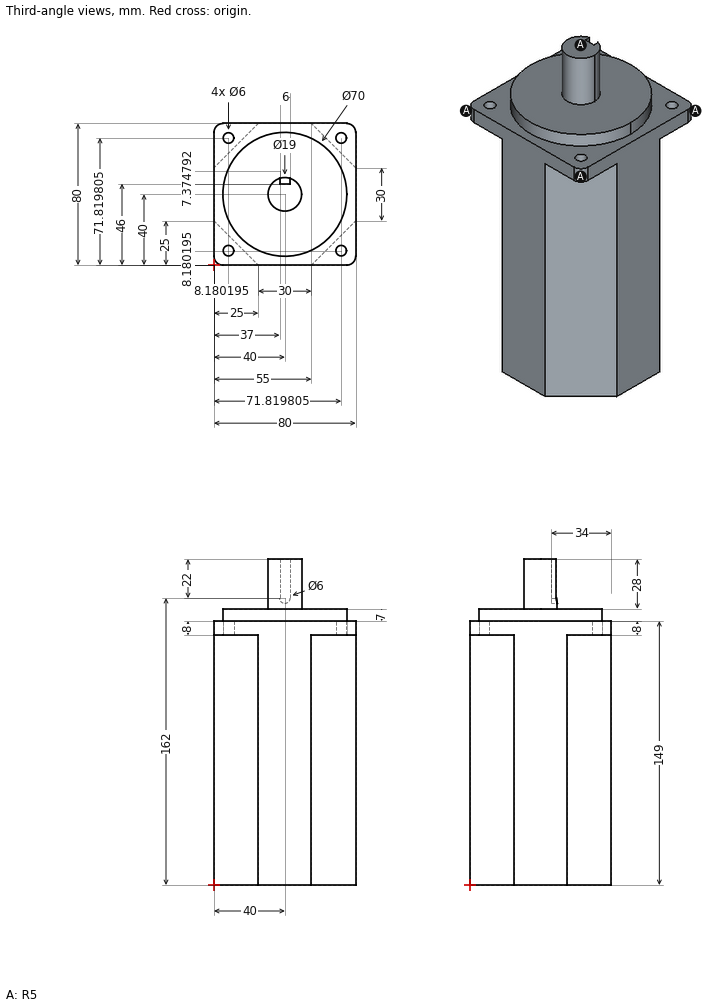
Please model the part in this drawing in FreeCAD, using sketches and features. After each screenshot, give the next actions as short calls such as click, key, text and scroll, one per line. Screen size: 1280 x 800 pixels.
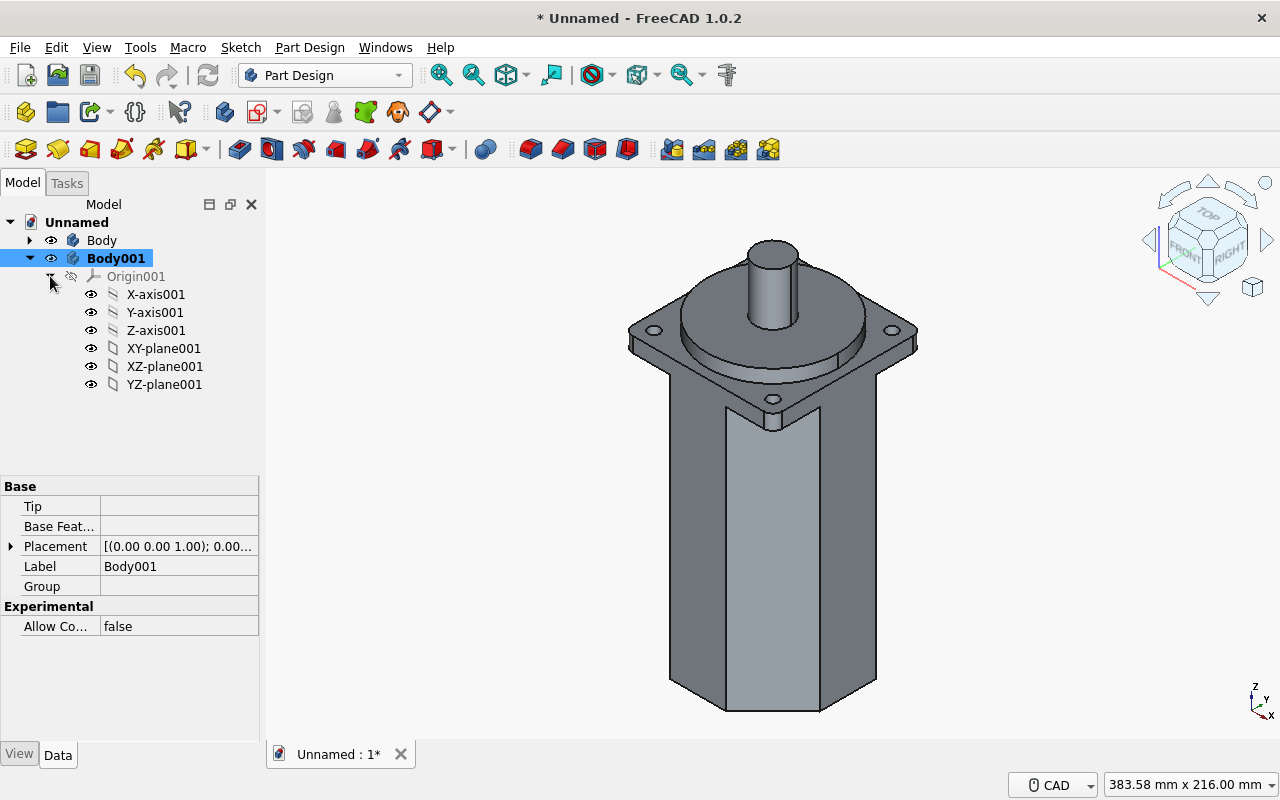
click(136, 348)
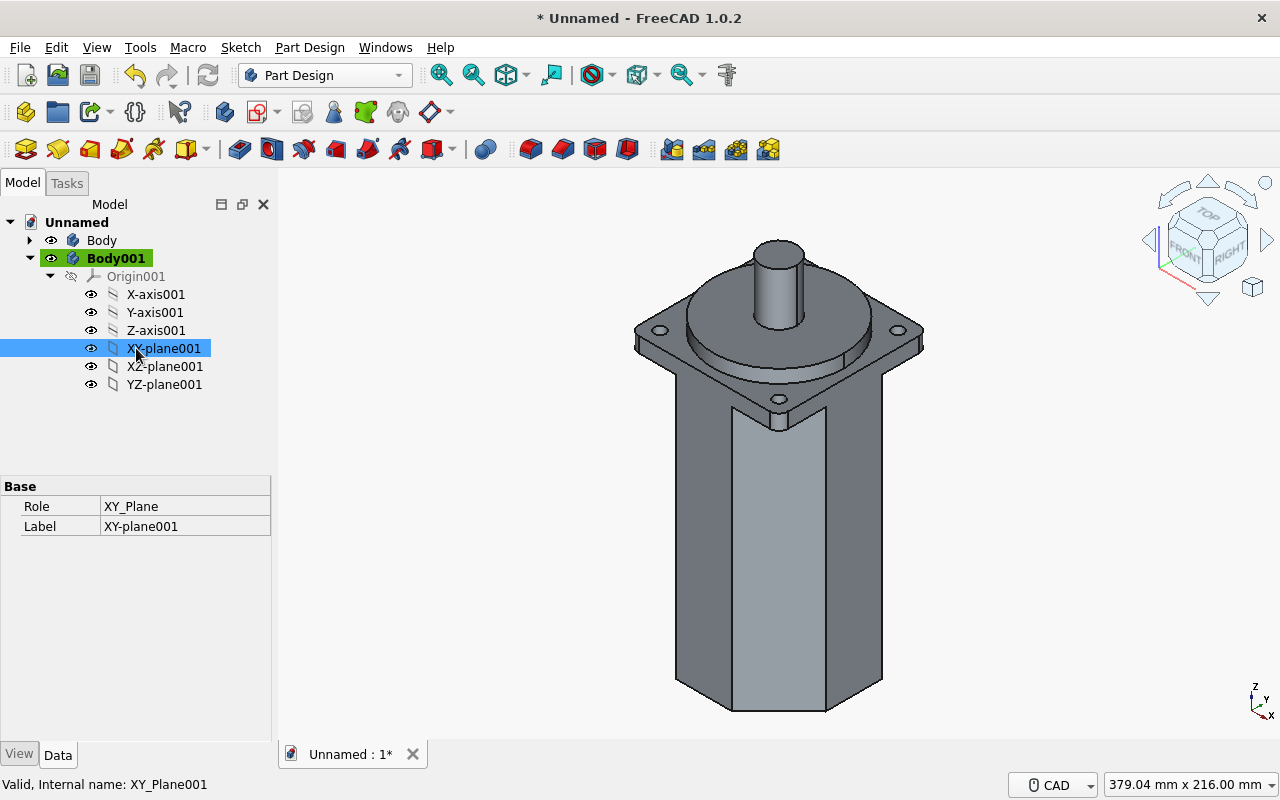
click(430, 112)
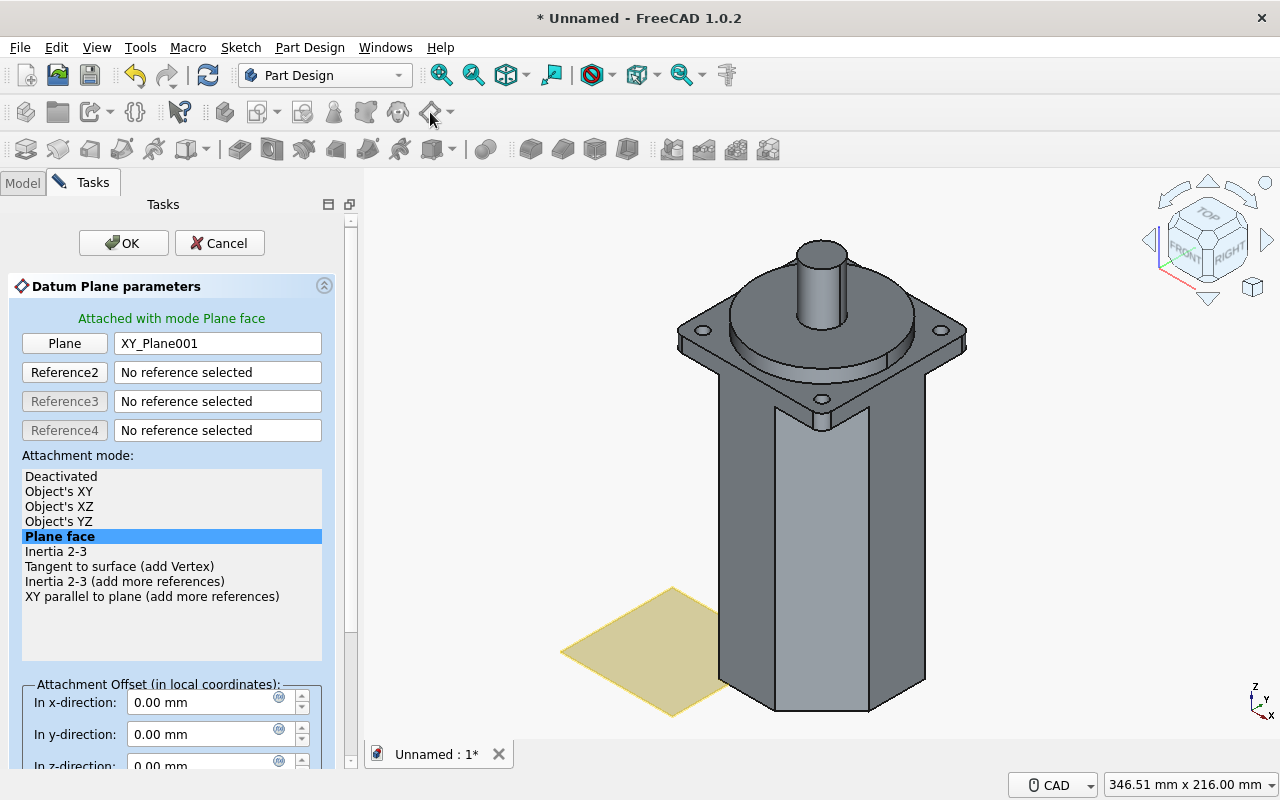
scroll(351, 491, down, 2)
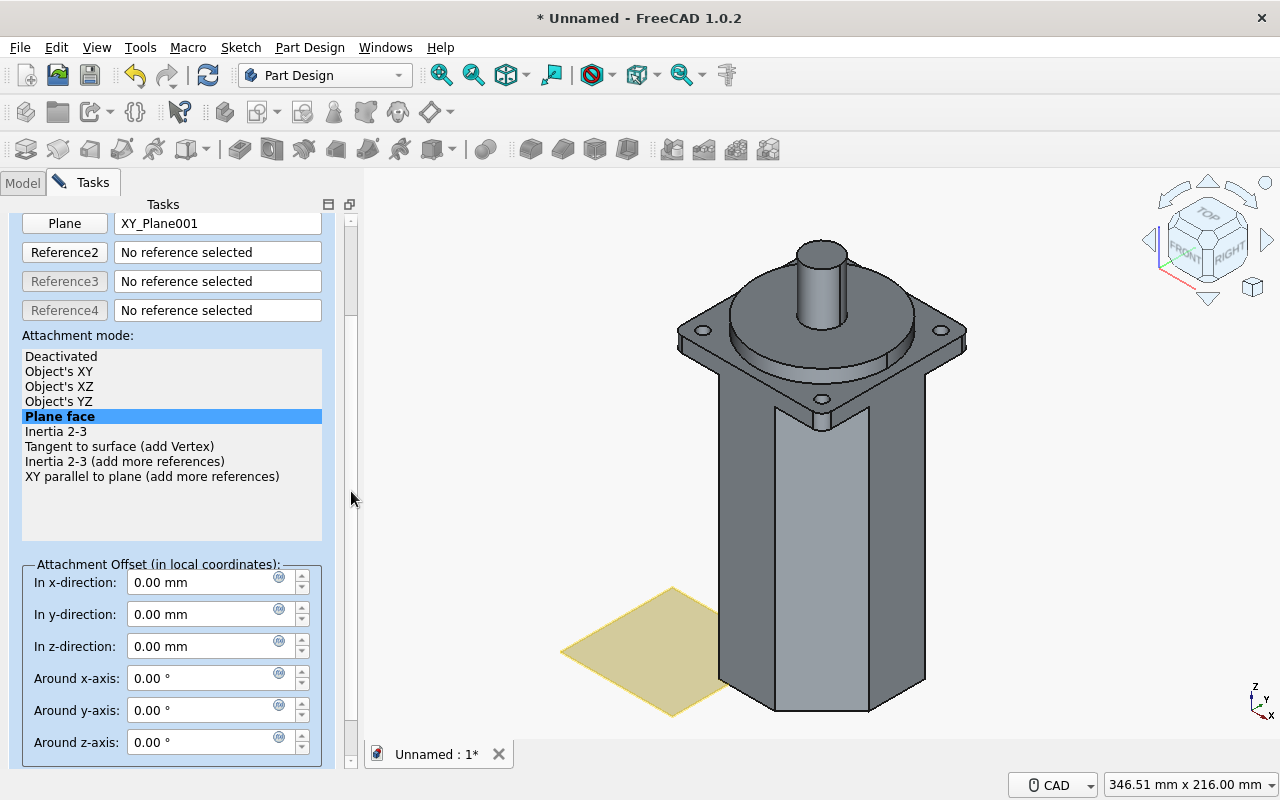
triple_click(210, 646)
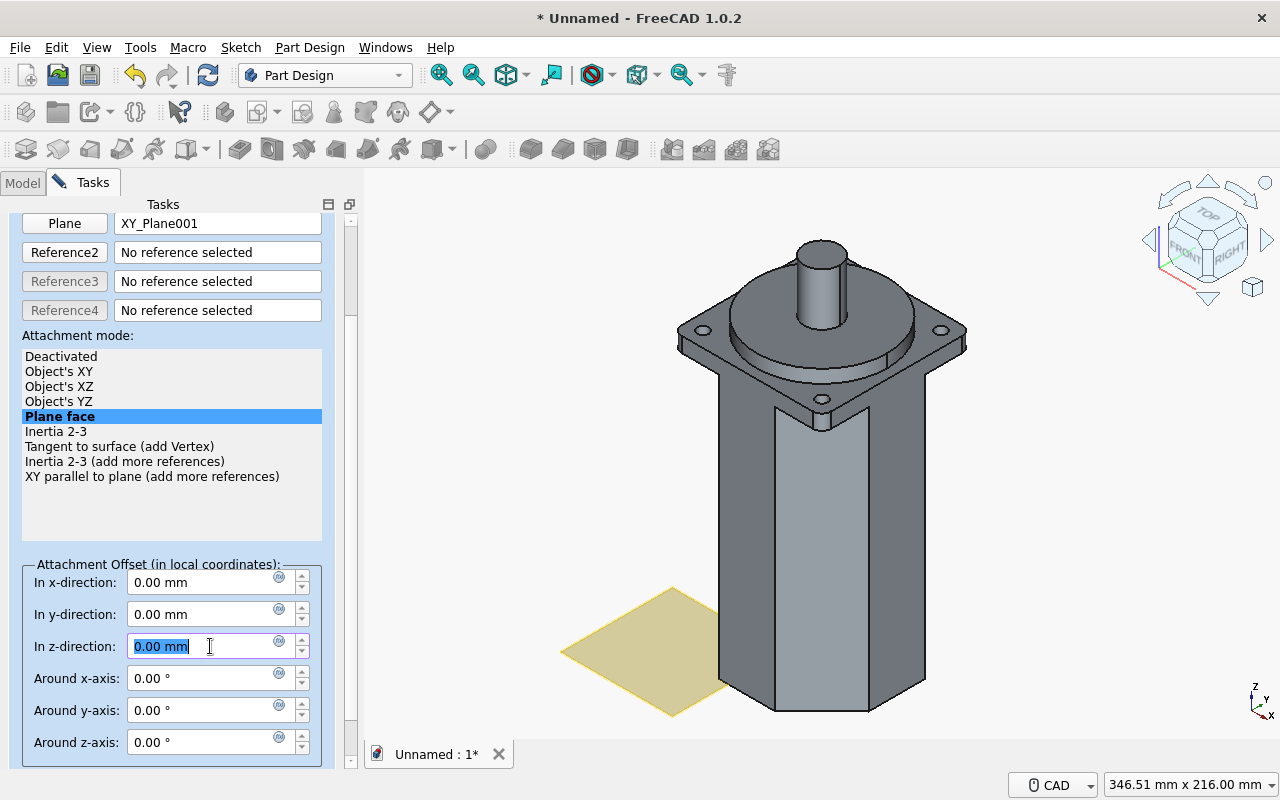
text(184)
key(Tab)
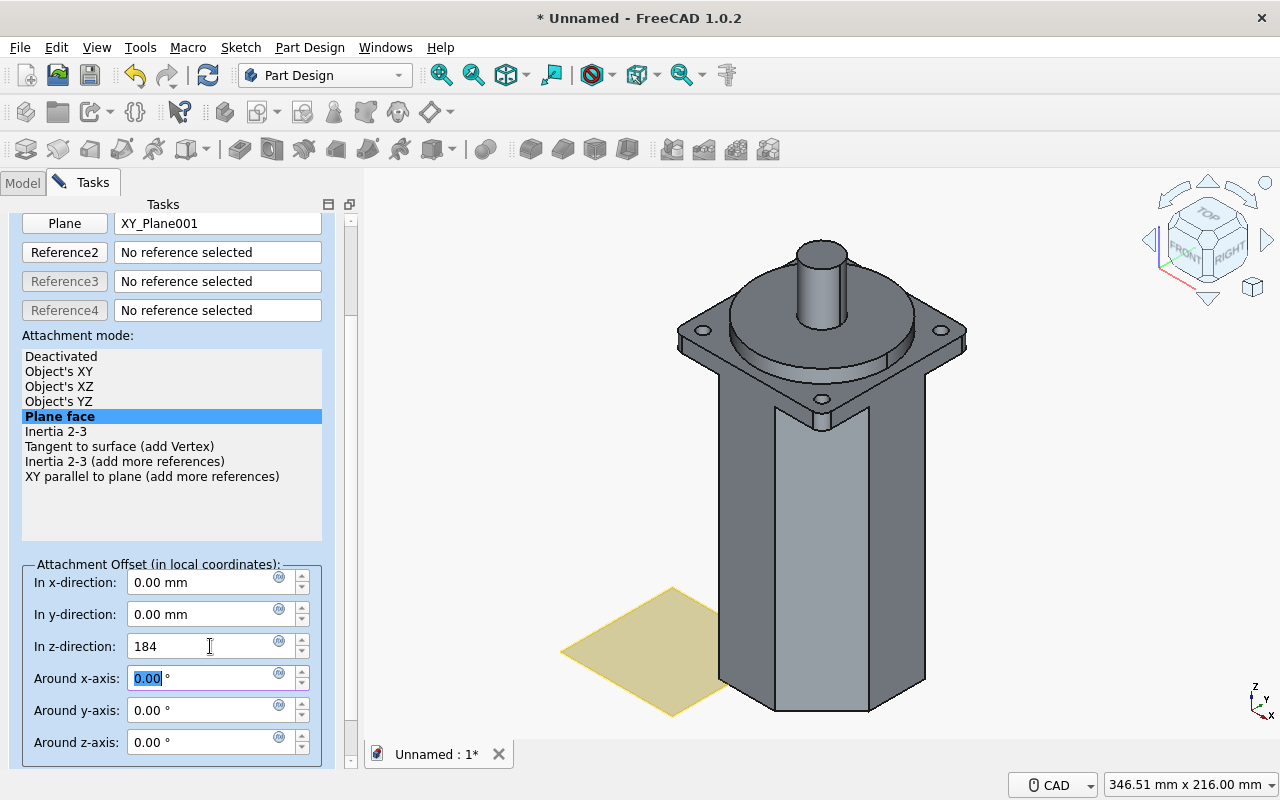
scroll(351, 491, up, 3)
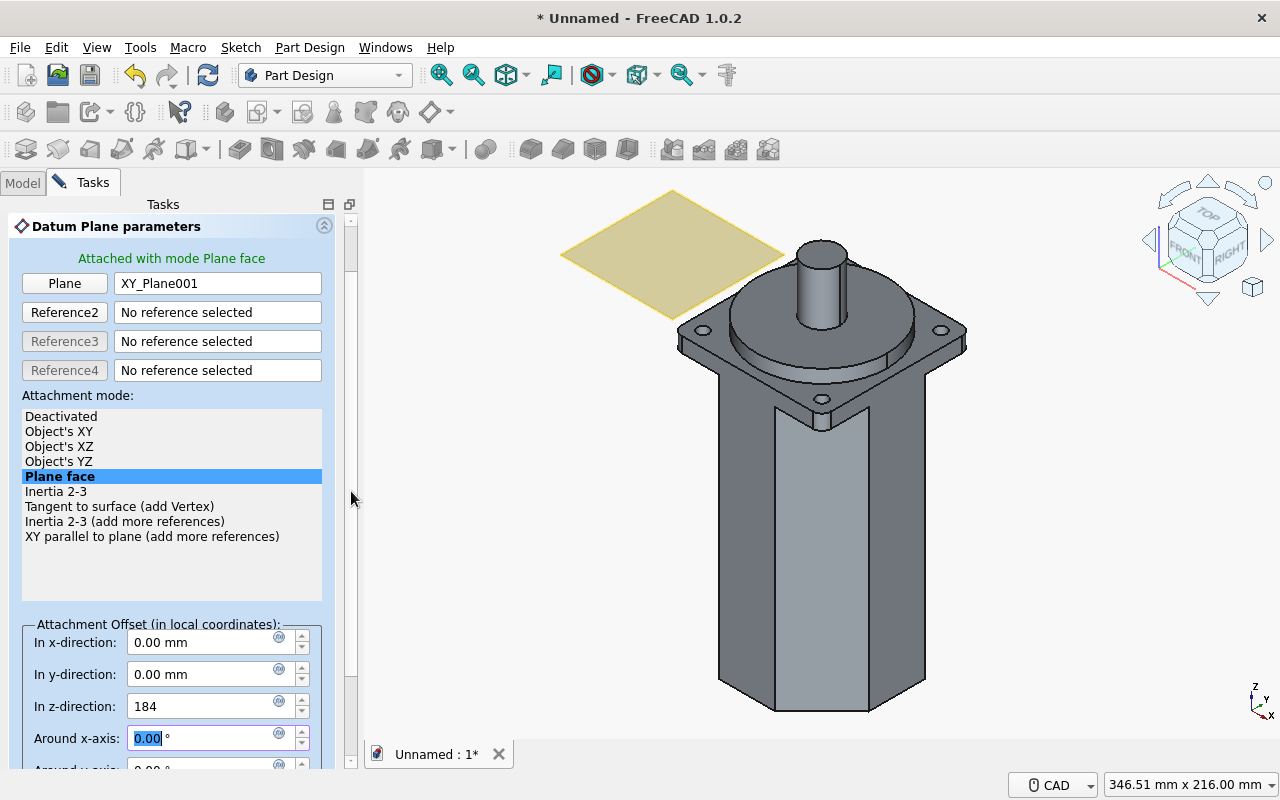
click(124, 243)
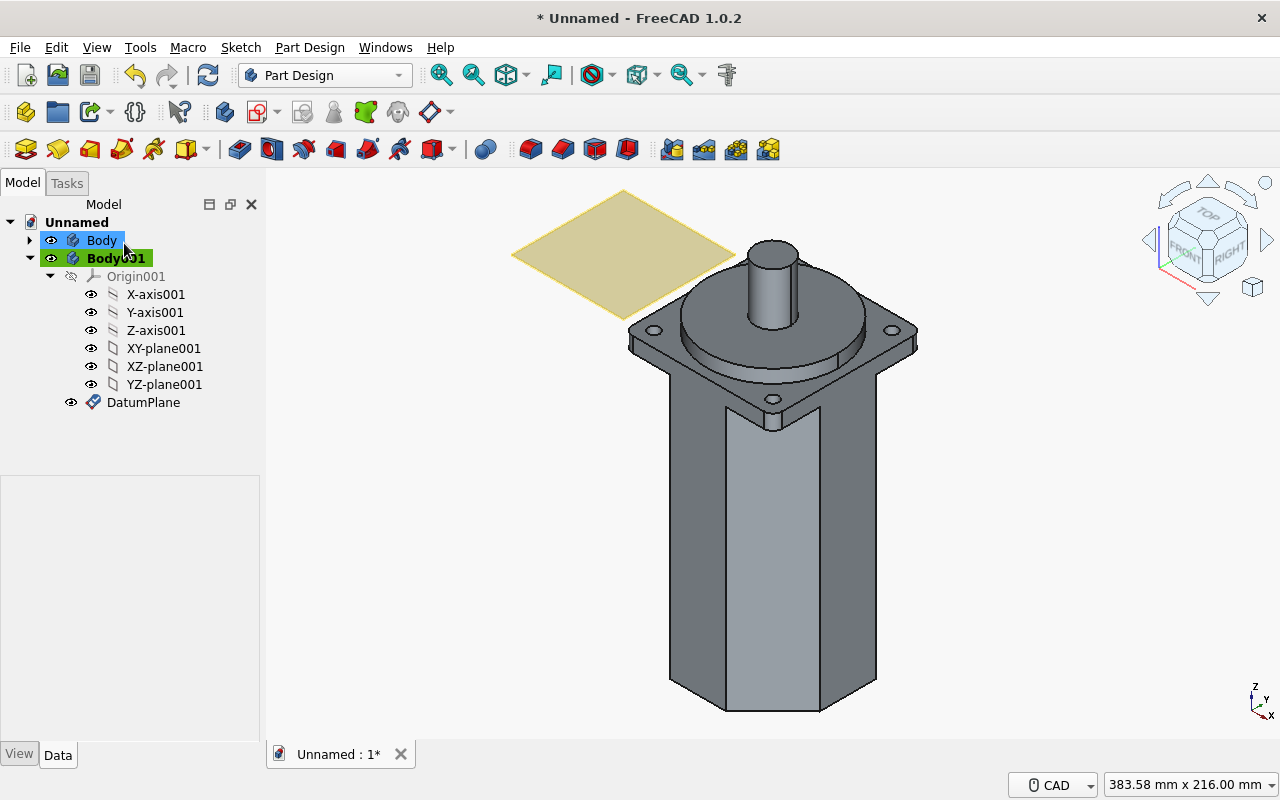
click(116, 402)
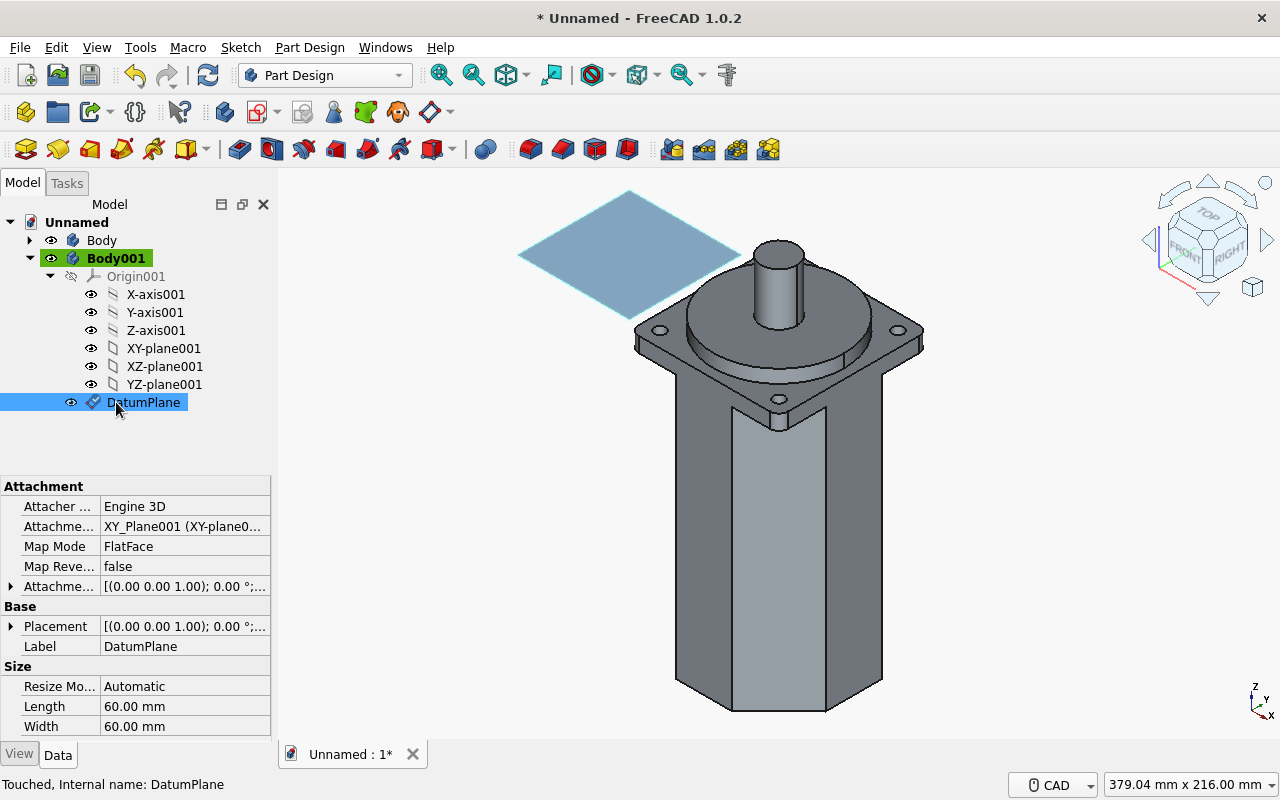
click(258, 112)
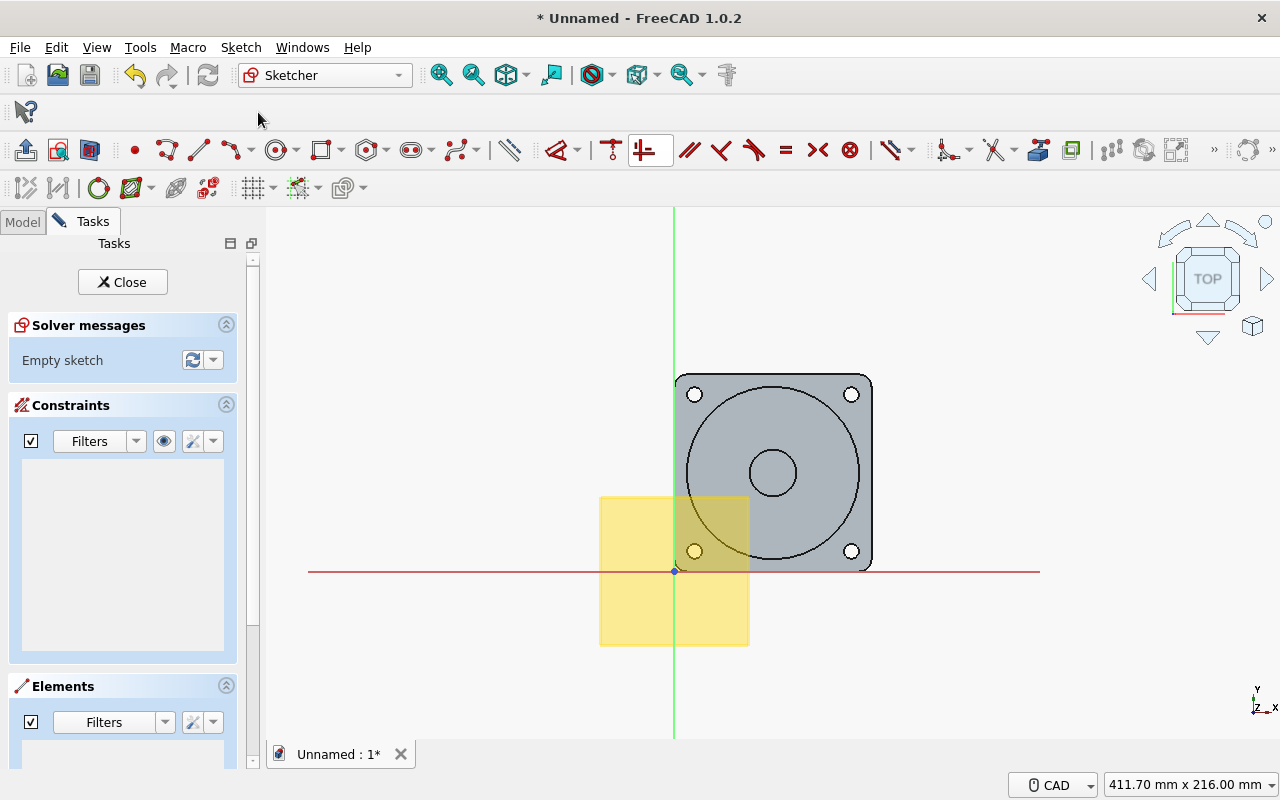
scroll(777, 448, up, 15)